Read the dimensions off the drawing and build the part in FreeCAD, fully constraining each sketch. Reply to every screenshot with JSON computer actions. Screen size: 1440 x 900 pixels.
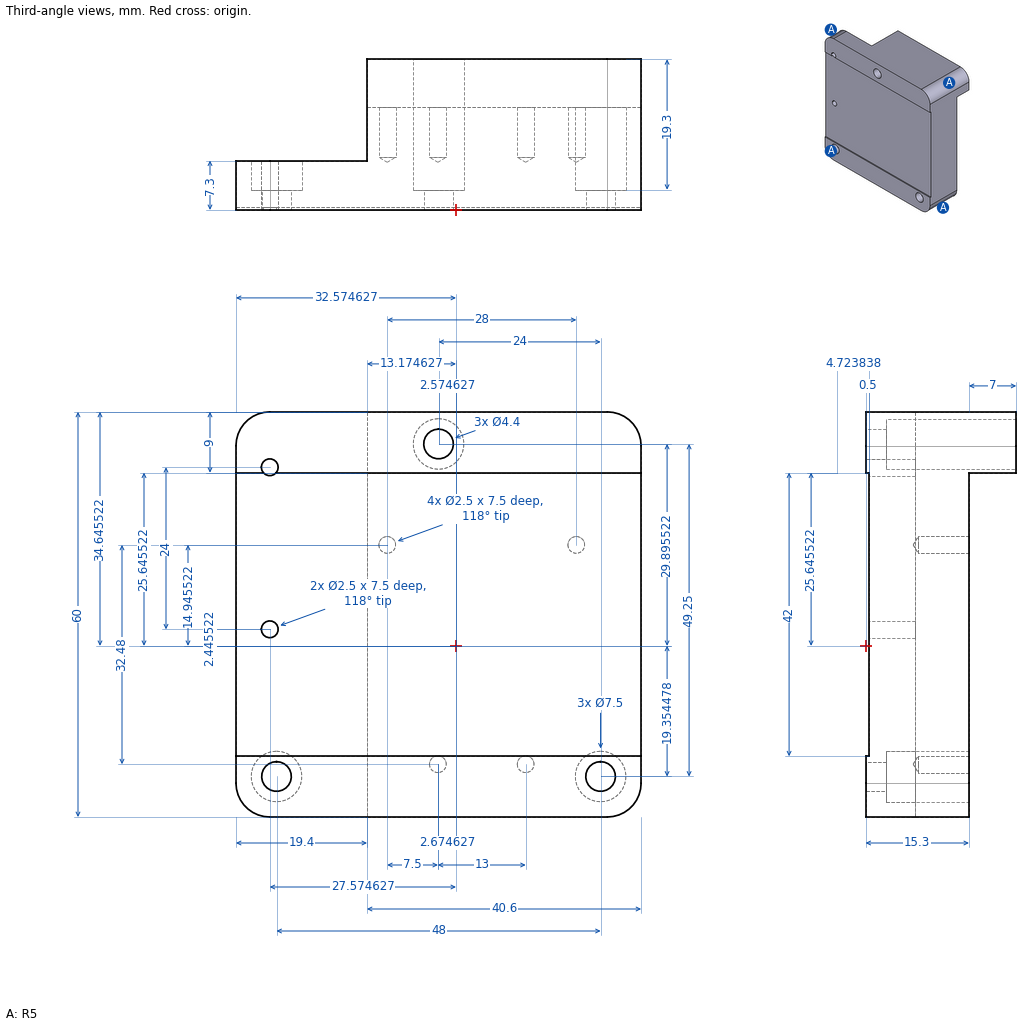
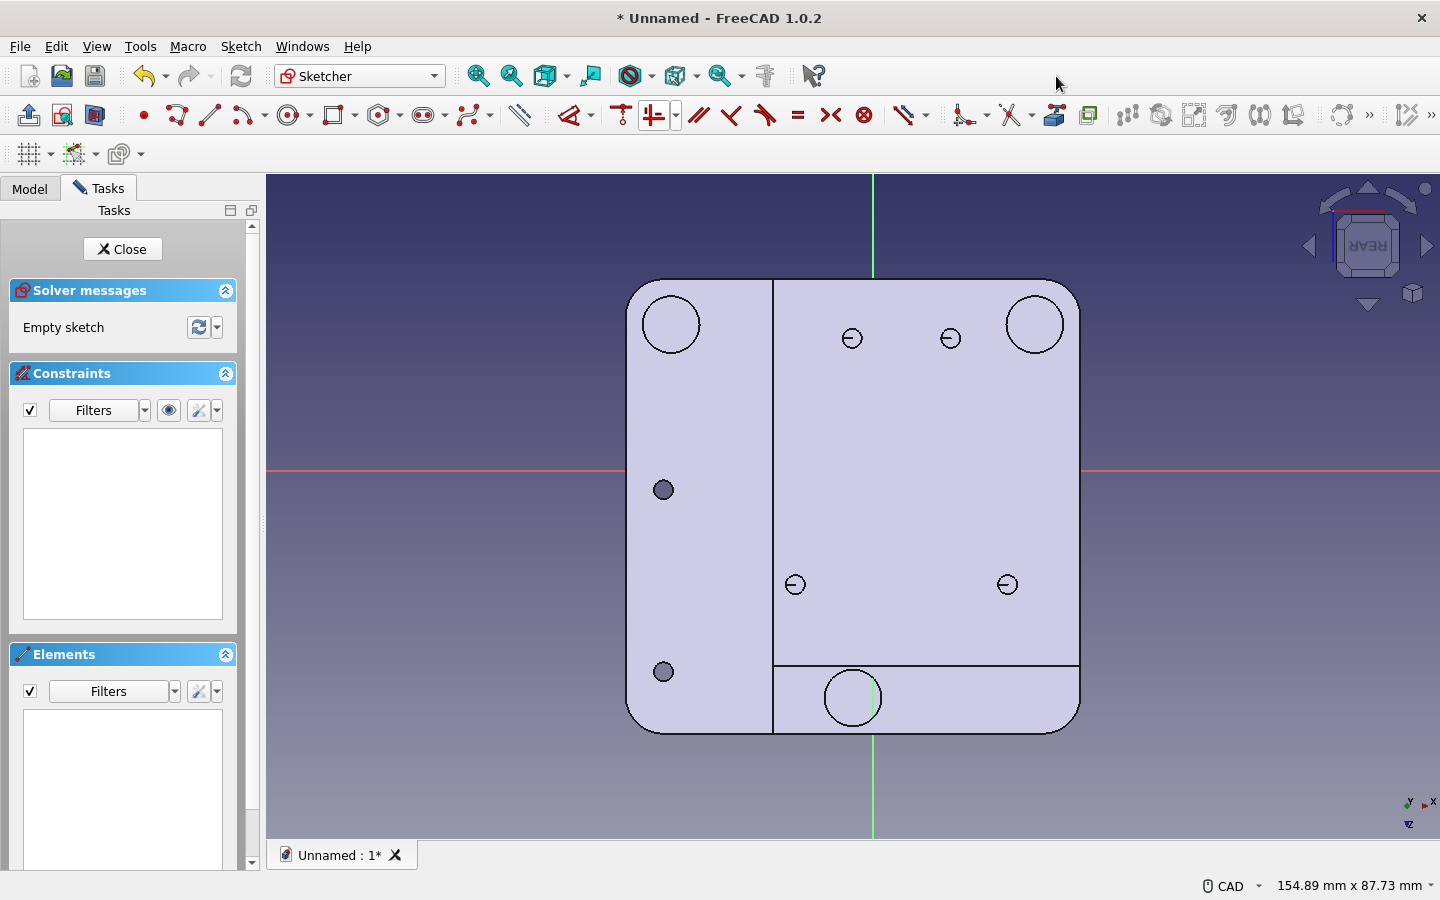
{"action": "left_click", "coordinate": [95, 116]}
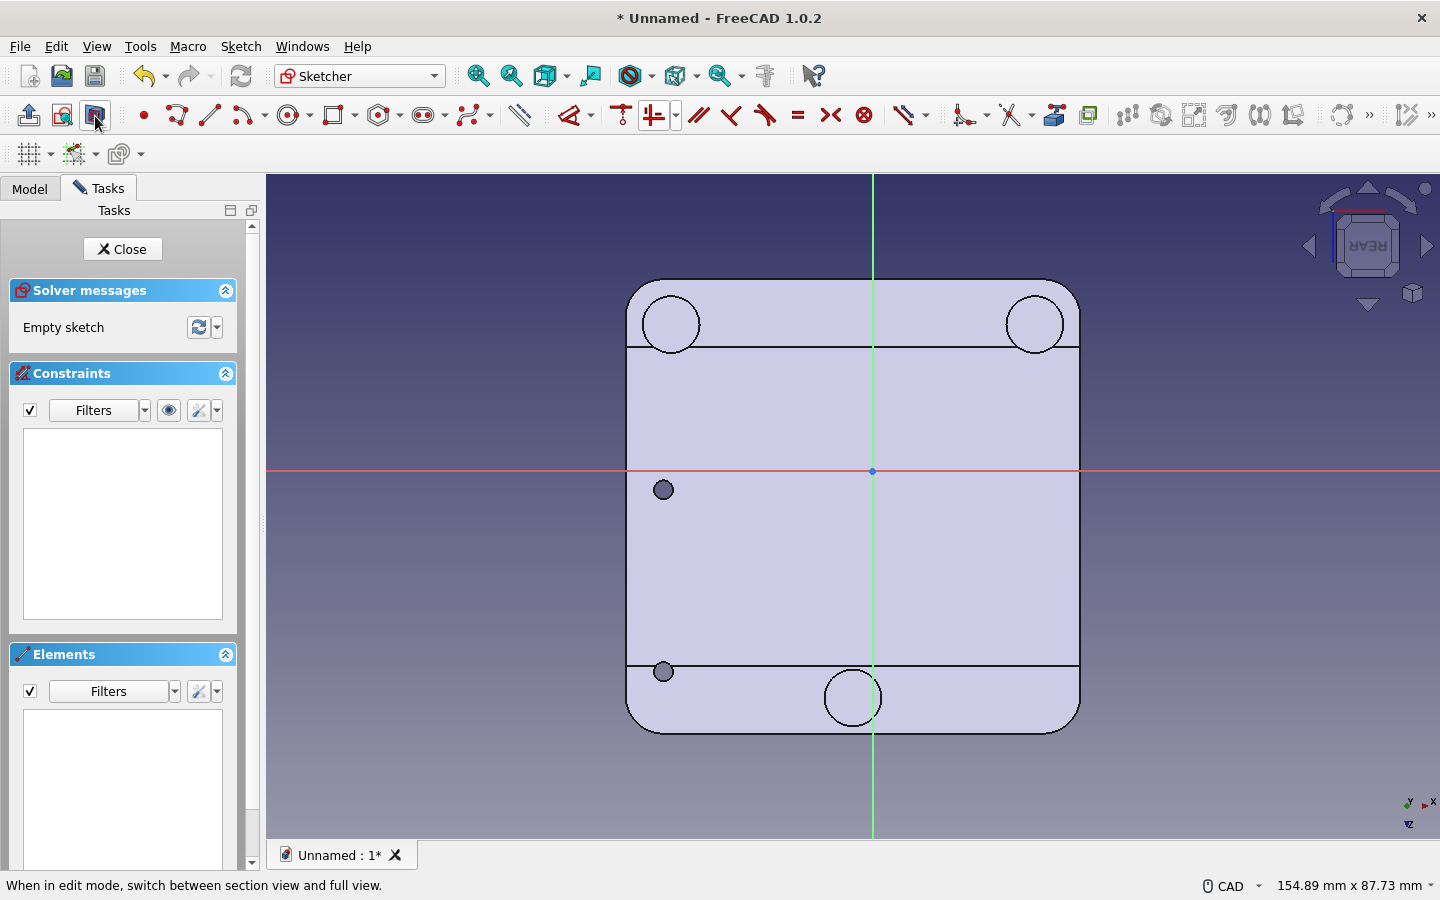
{"action": "key", "text": "g c"}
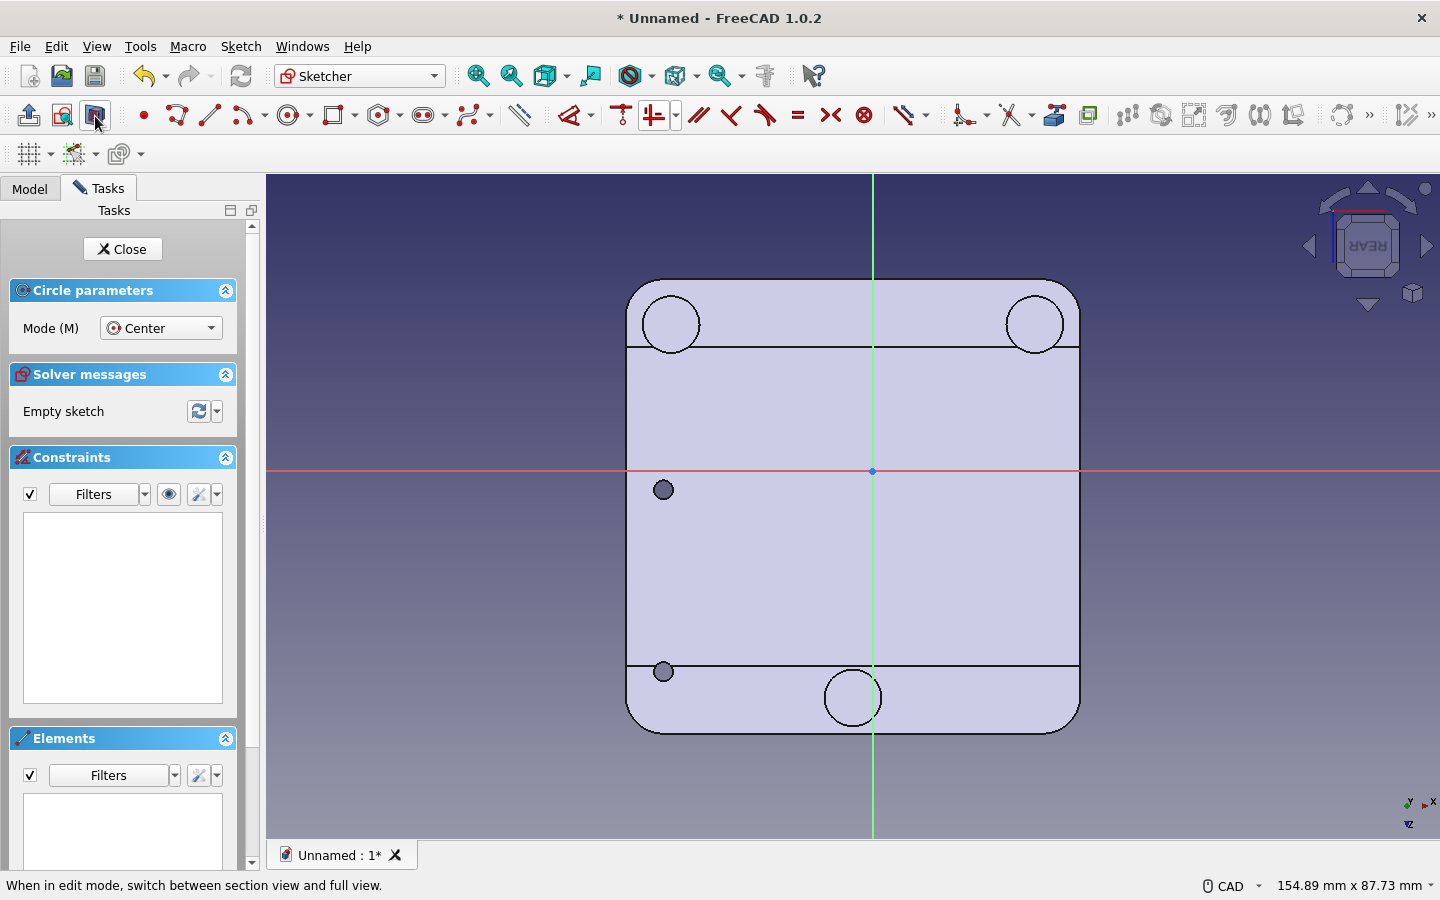
{"action": "scroll", "coordinate": [853, 698], "scroll_direction": "up", "scroll_amount": 2}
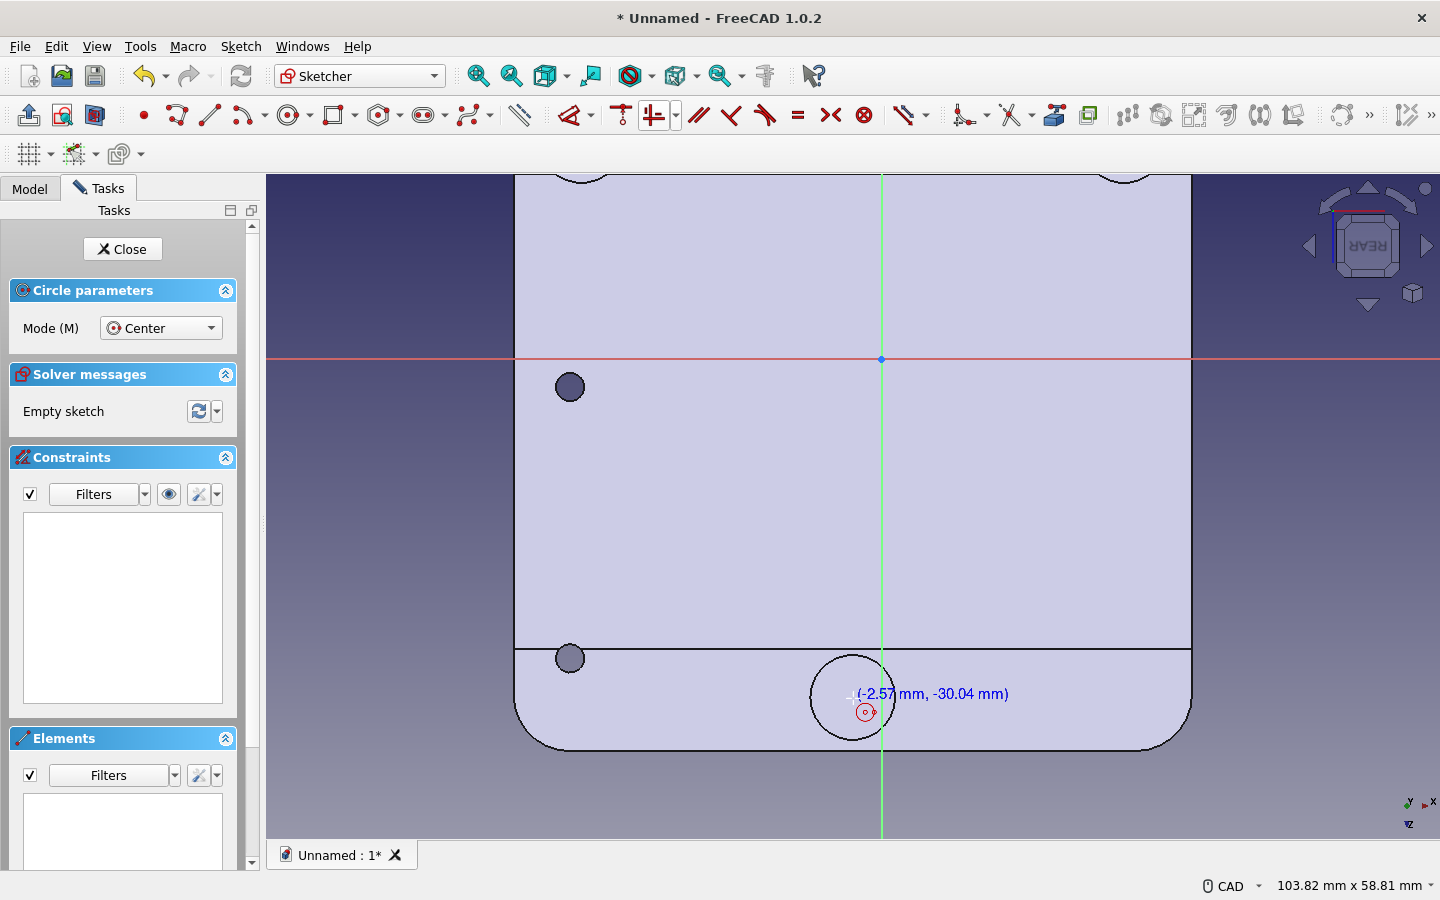
{"action": "left_click", "coordinate": [853, 697]}
{"action": "left_click", "coordinate": [835, 680]}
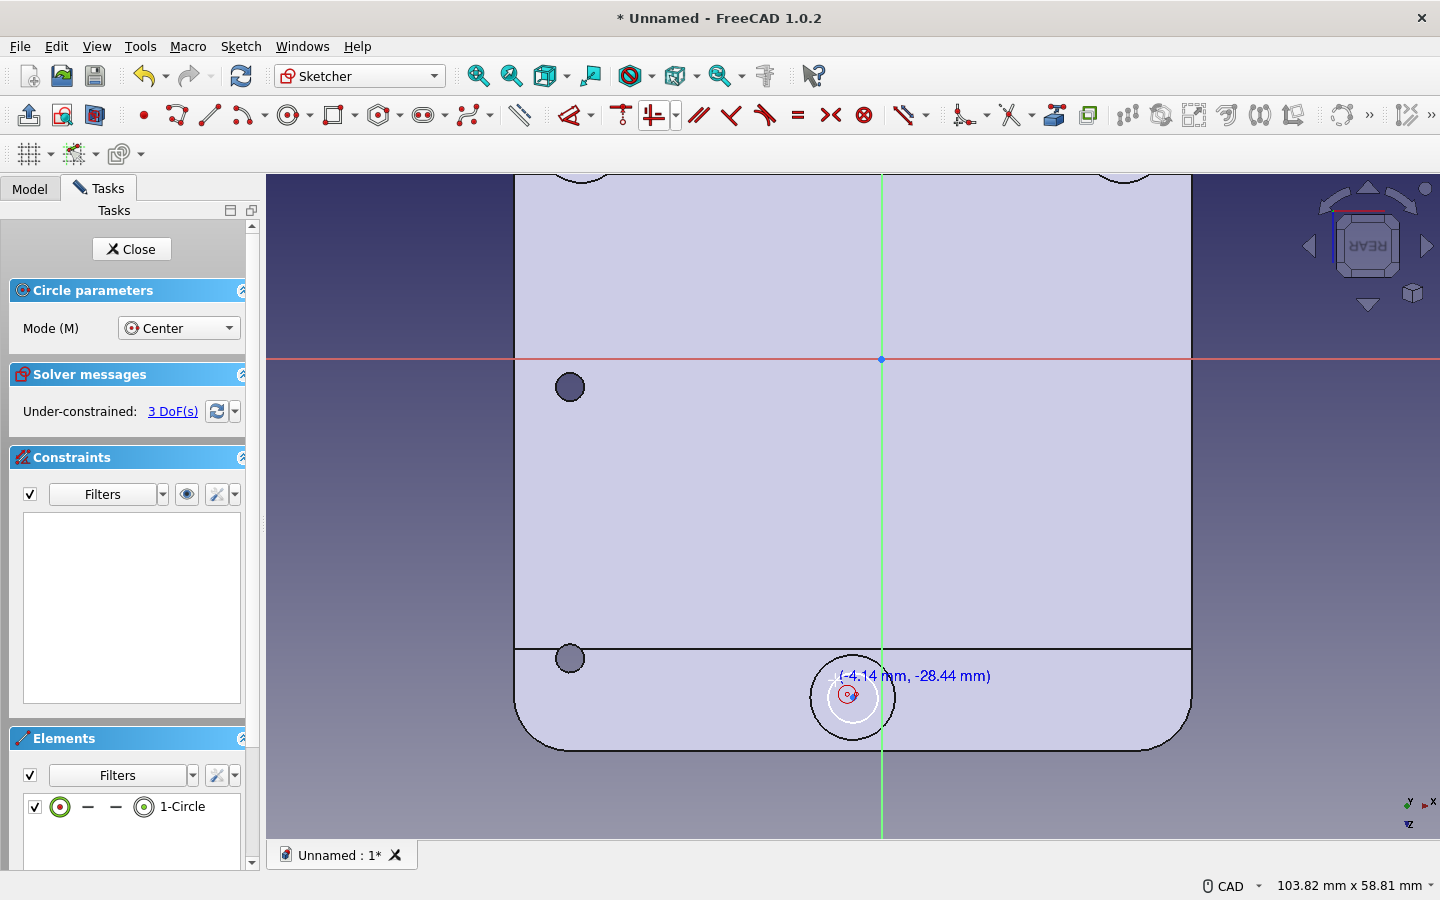
{"action": "scroll", "coordinate": [646, 684], "scroll_direction": "down", "scroll_amount": 2}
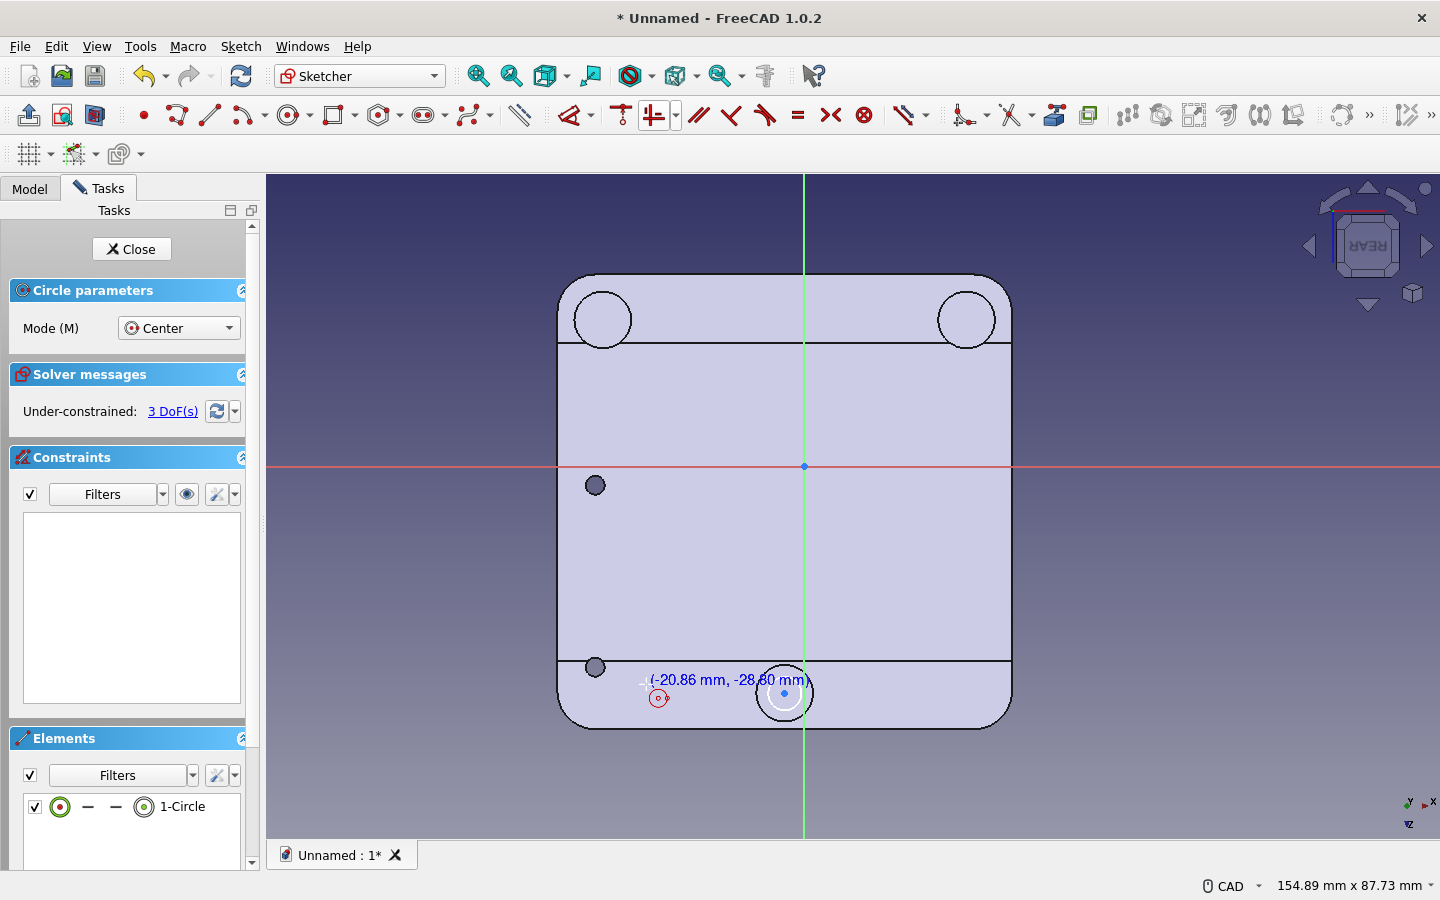
{"action": "scroll", "coordinate": [967, 320], "scroll_direction": "up", "scroll_amount": 2}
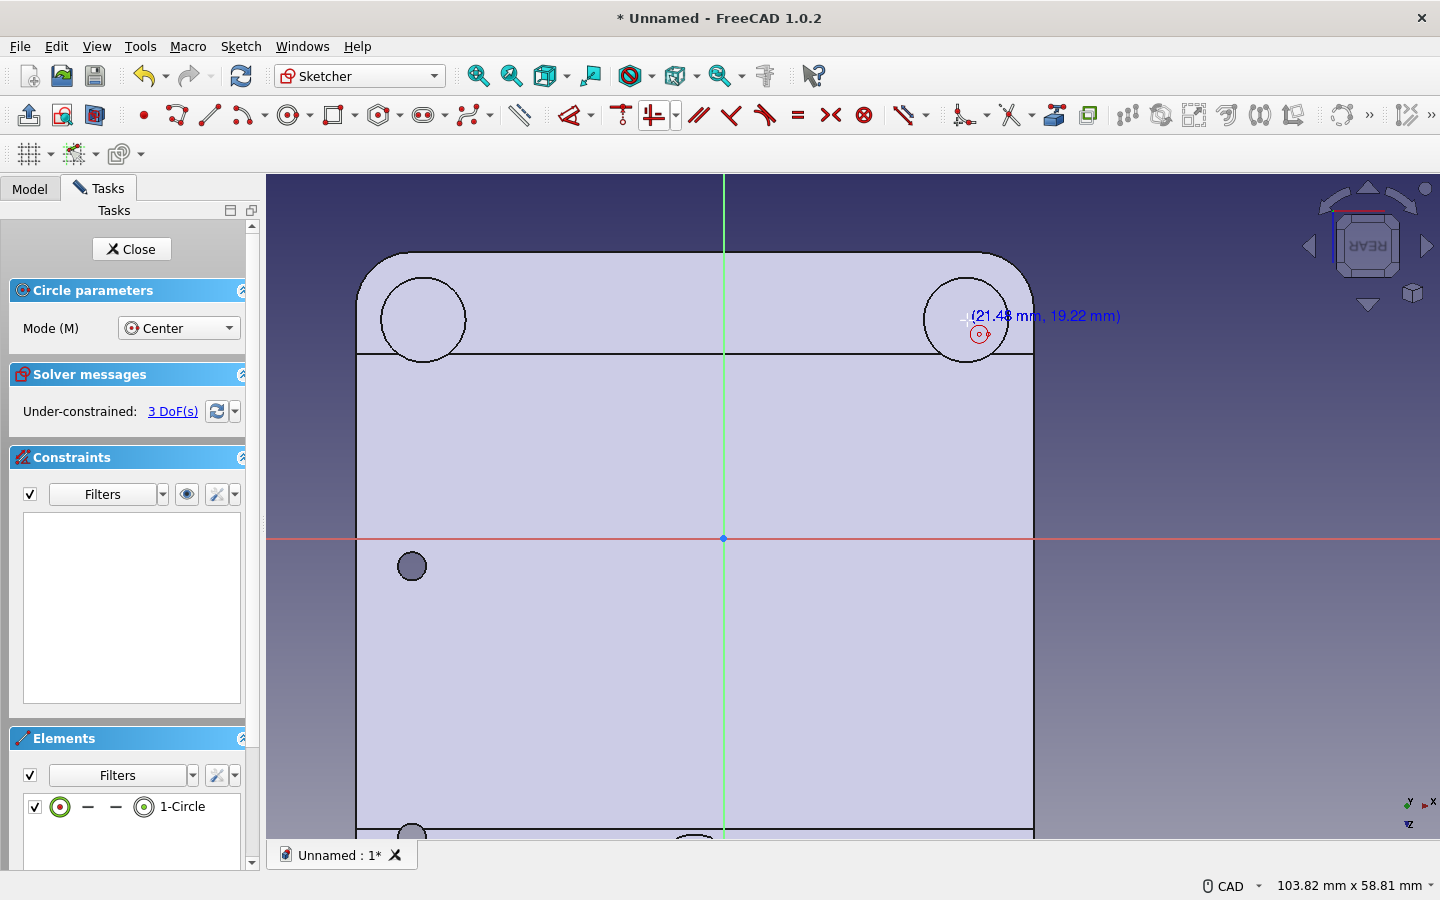
{"action": "left_click", "coordinate": [966, 320]}
{"action": "left_click", "coordinate": [984, 302]}